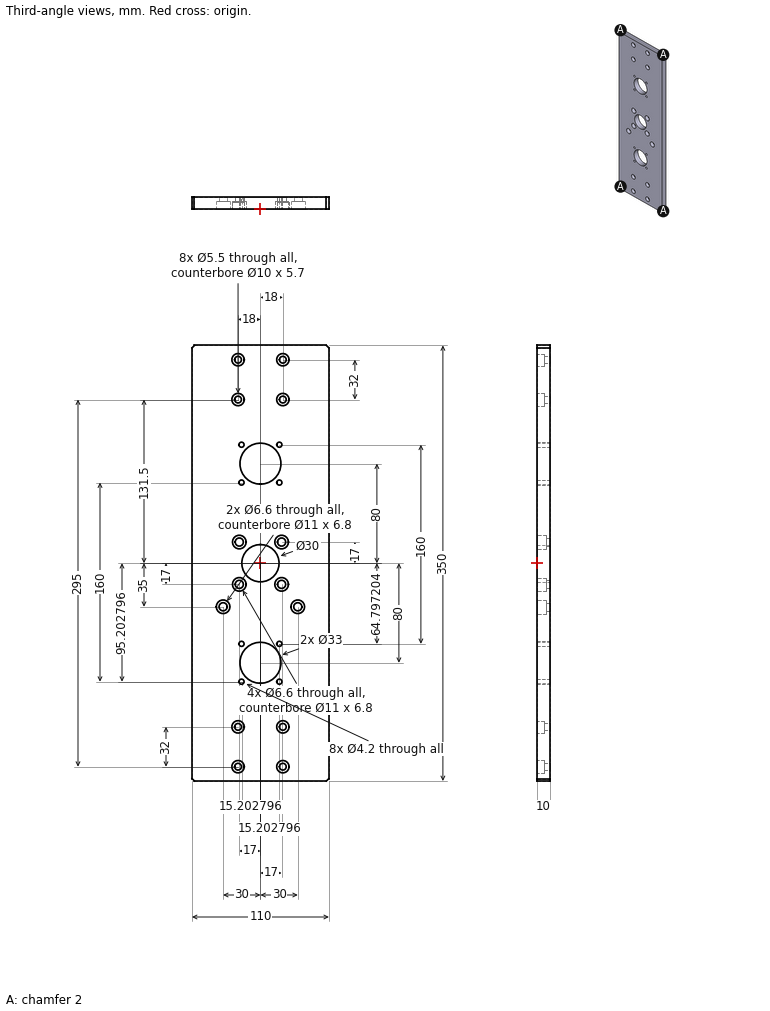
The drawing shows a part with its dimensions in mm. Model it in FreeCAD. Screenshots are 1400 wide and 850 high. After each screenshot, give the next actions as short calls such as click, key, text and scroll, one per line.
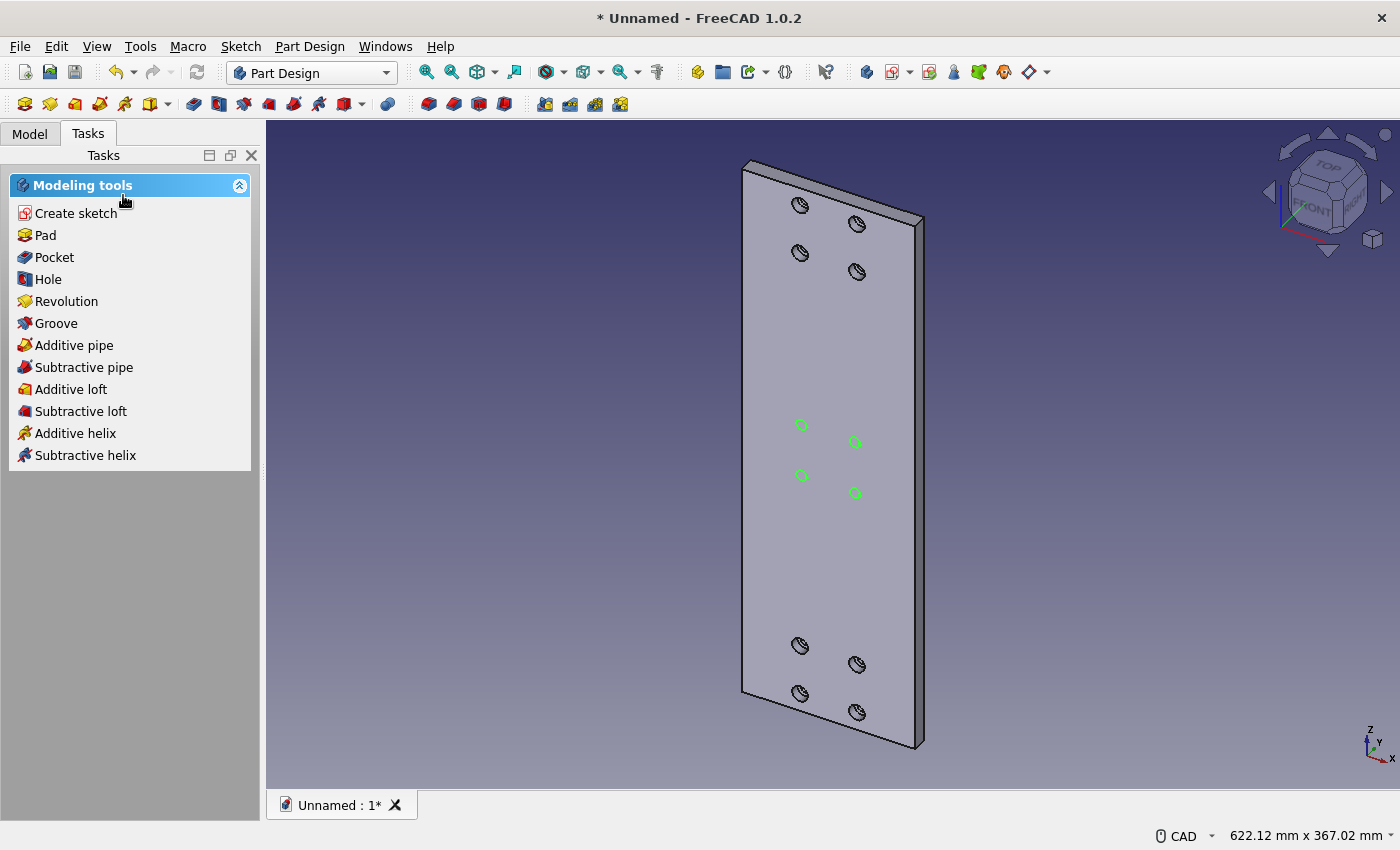
click(219, 104)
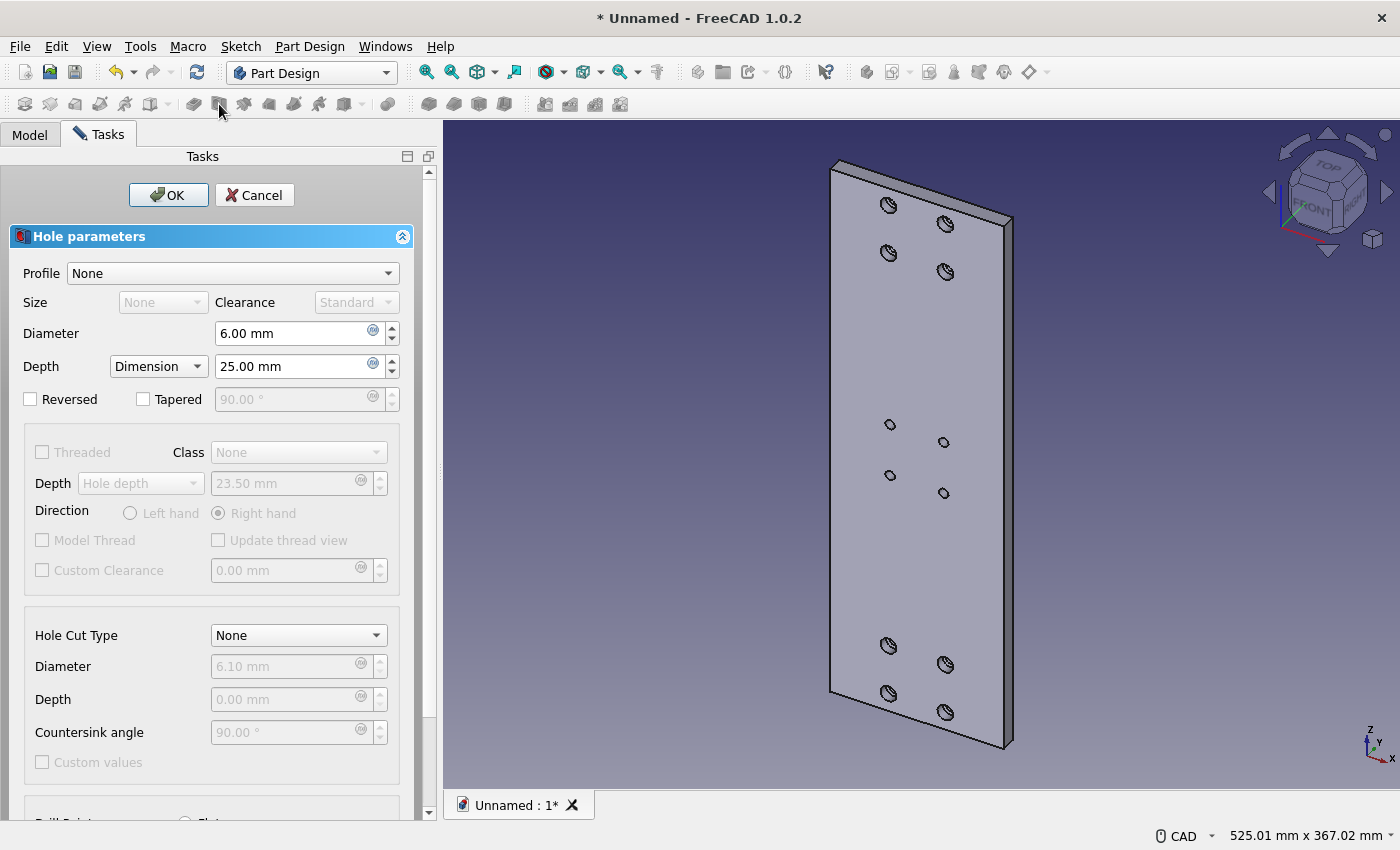
triple_click(300, 334)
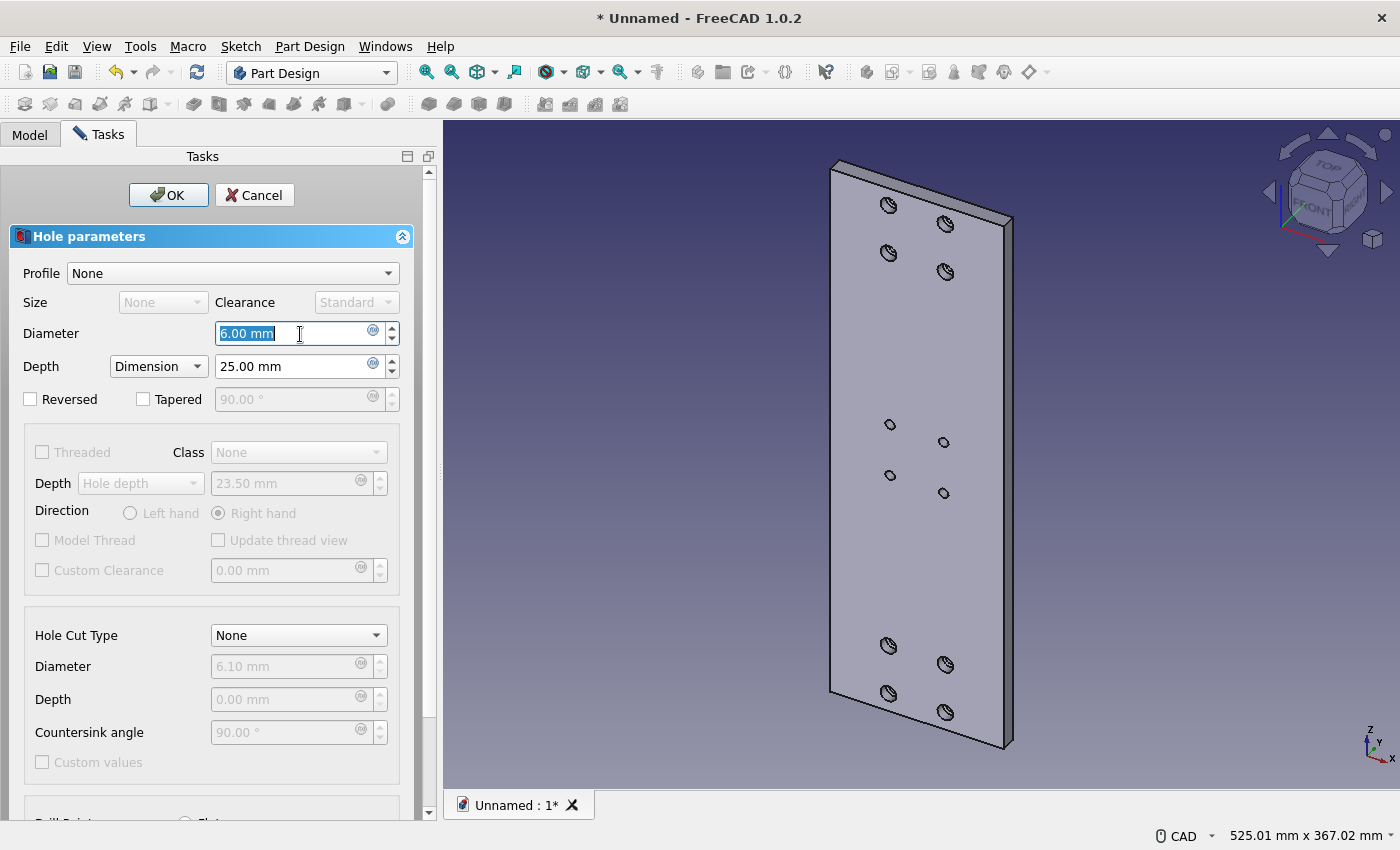
text(6.6)
key(Tab)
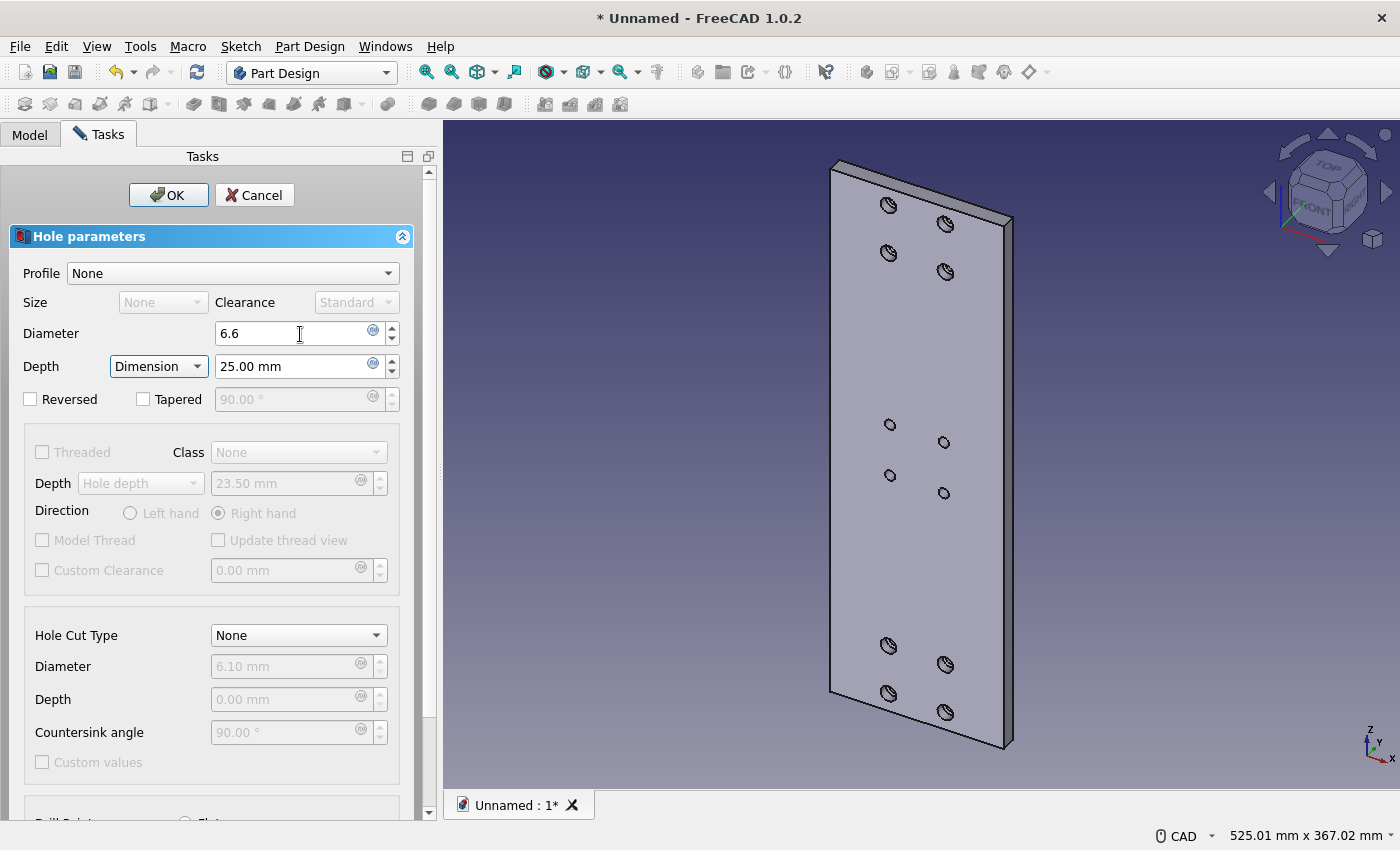
click(160, 366)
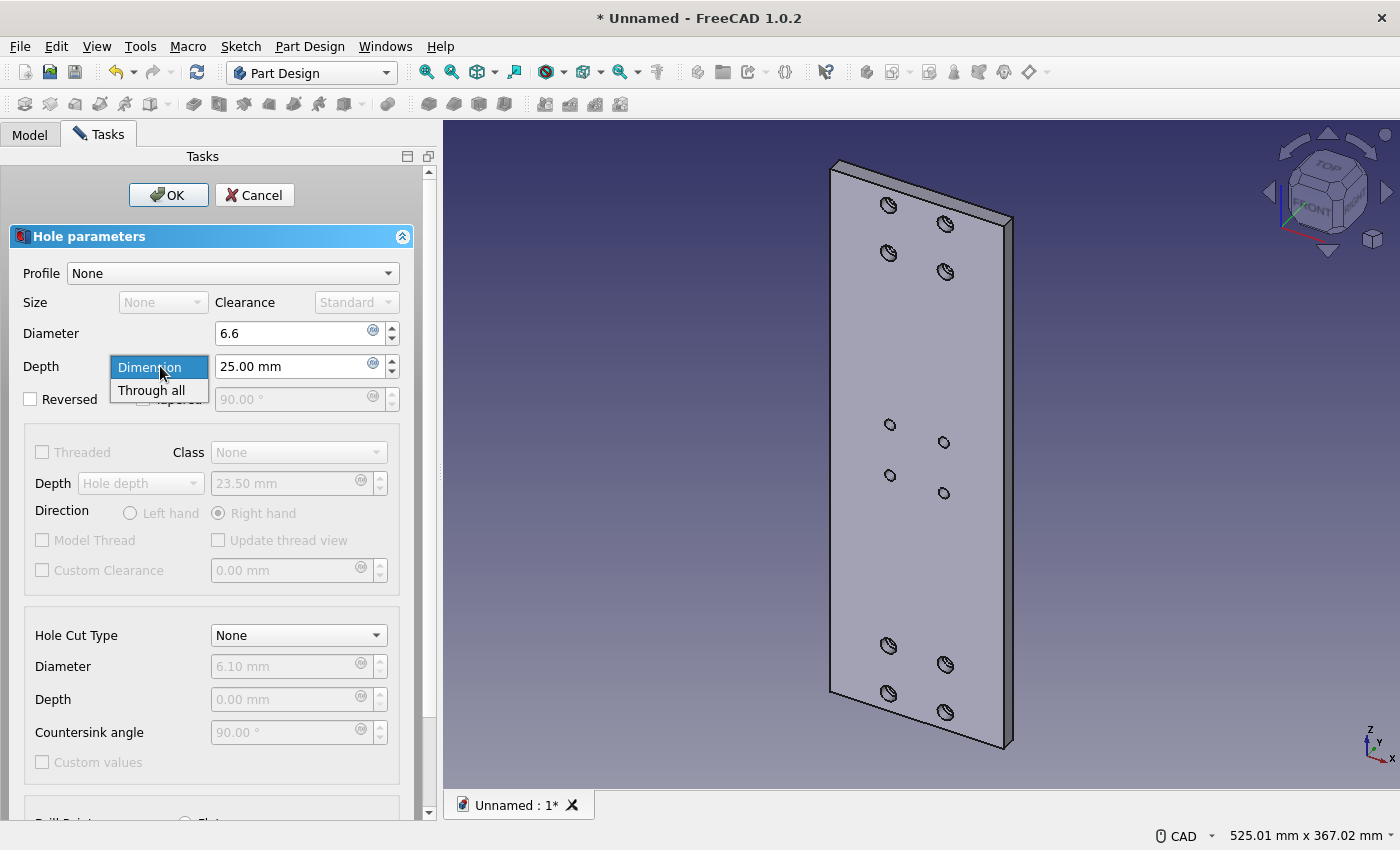
click(158, 390)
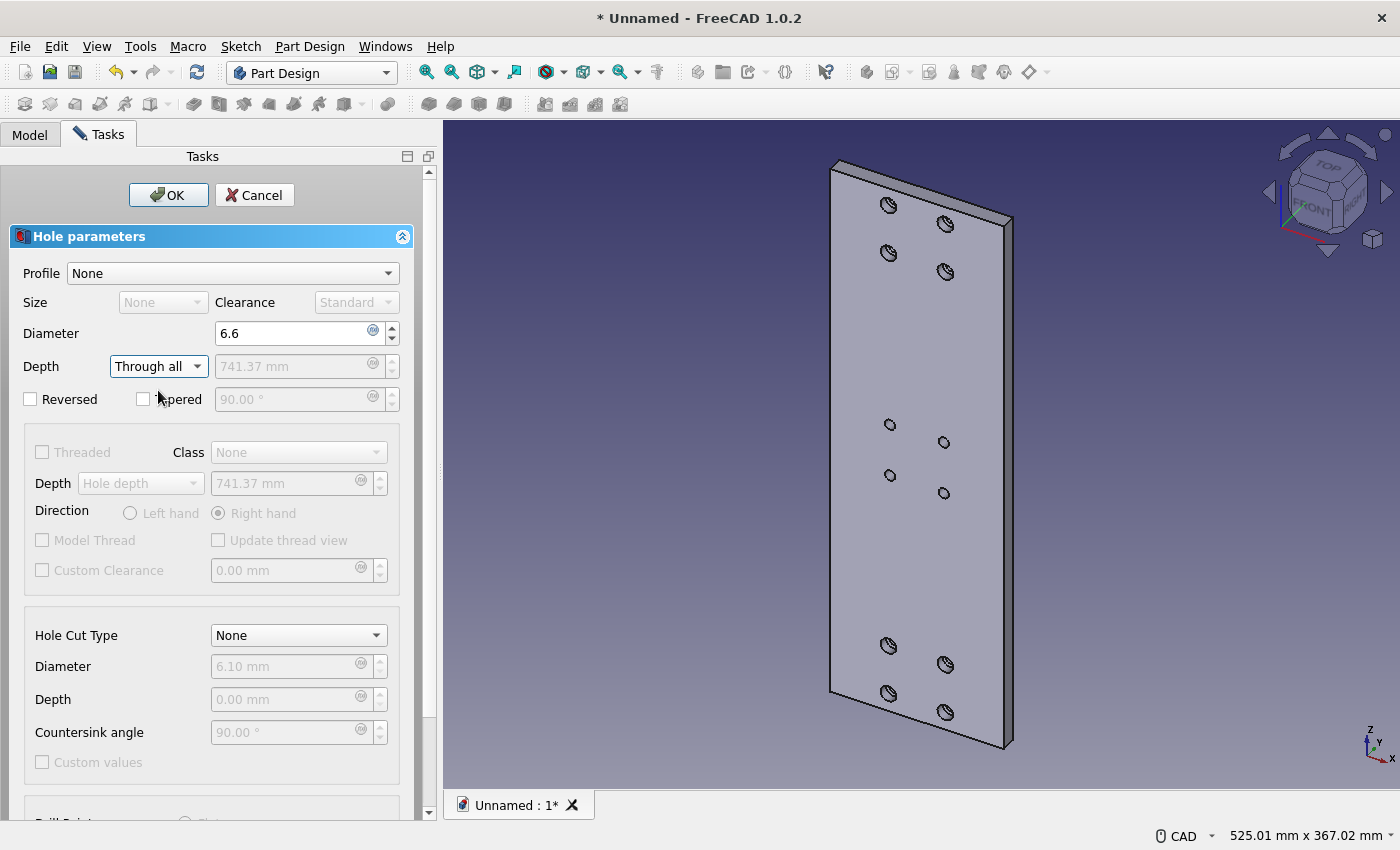
click(300, 636)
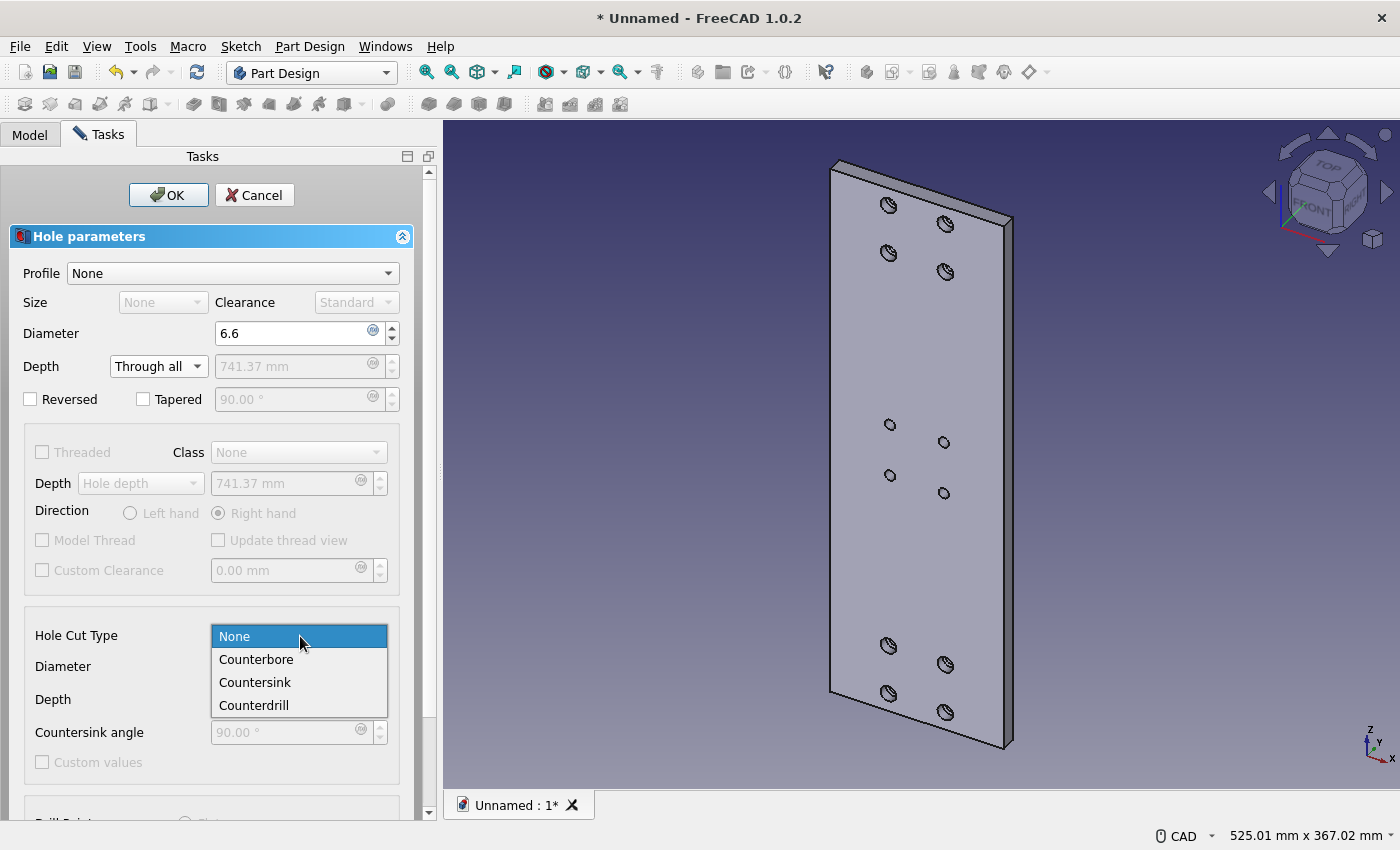
click(298, 660)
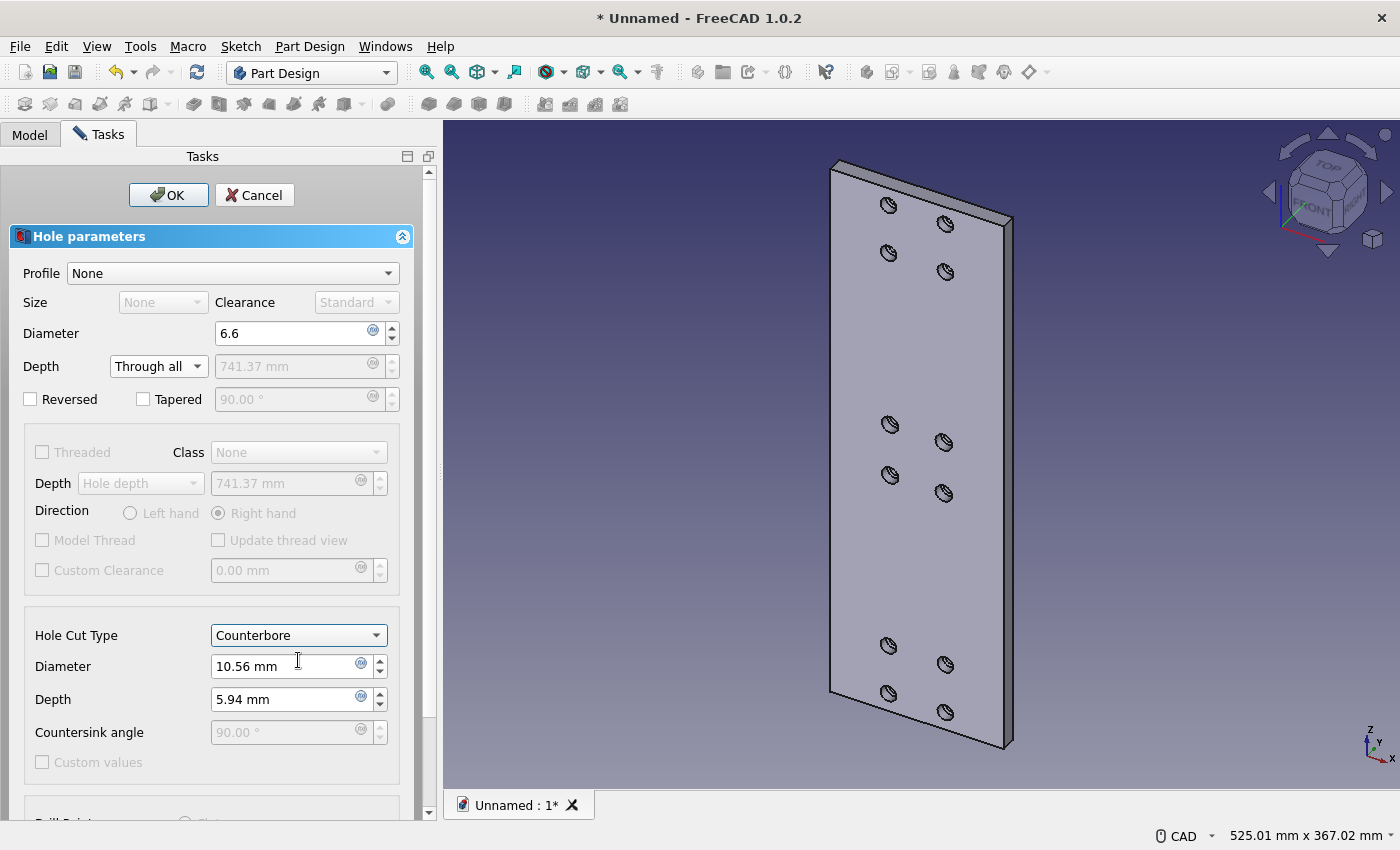
triple_click(292, 666)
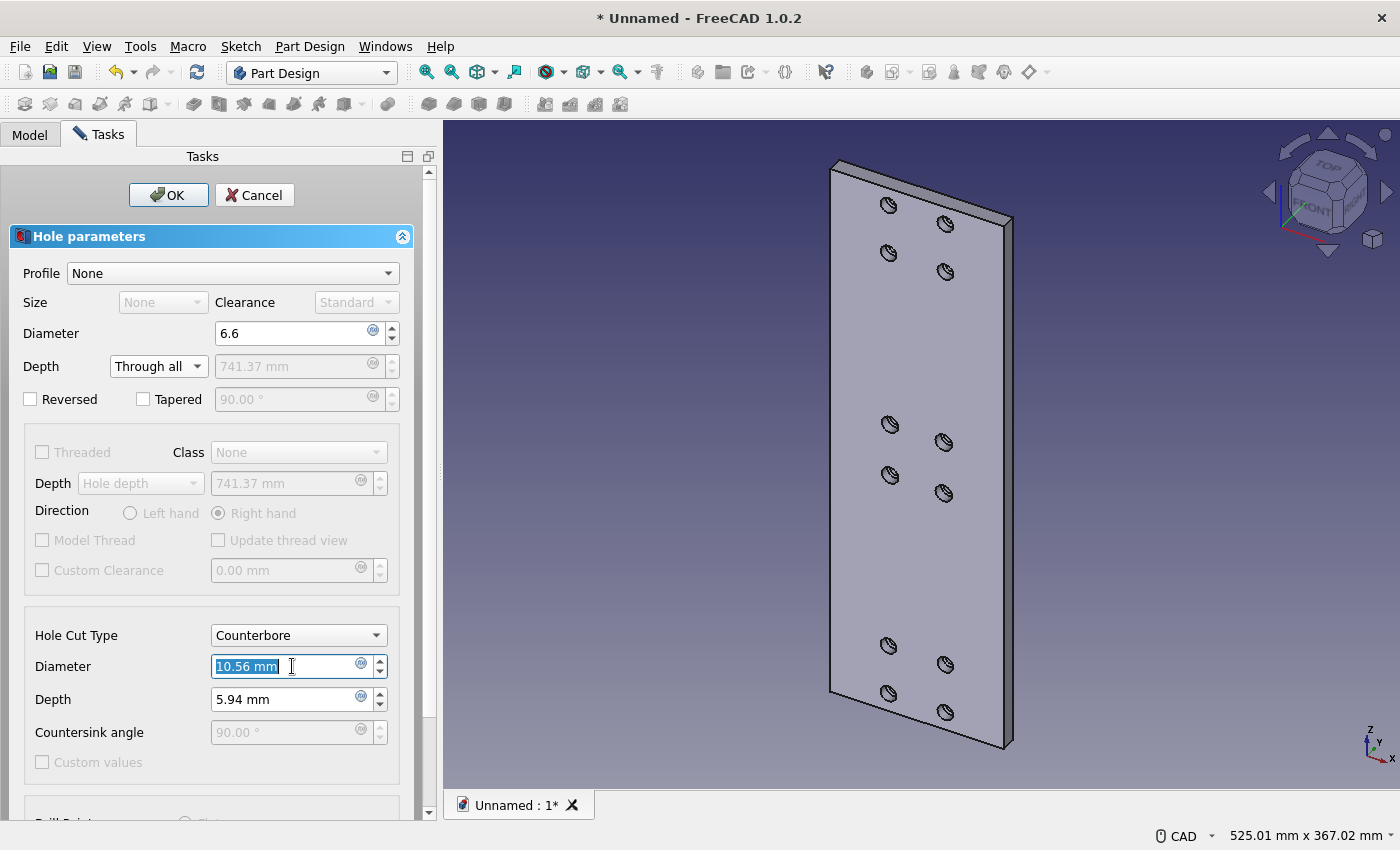
text(11)
key(Tab)